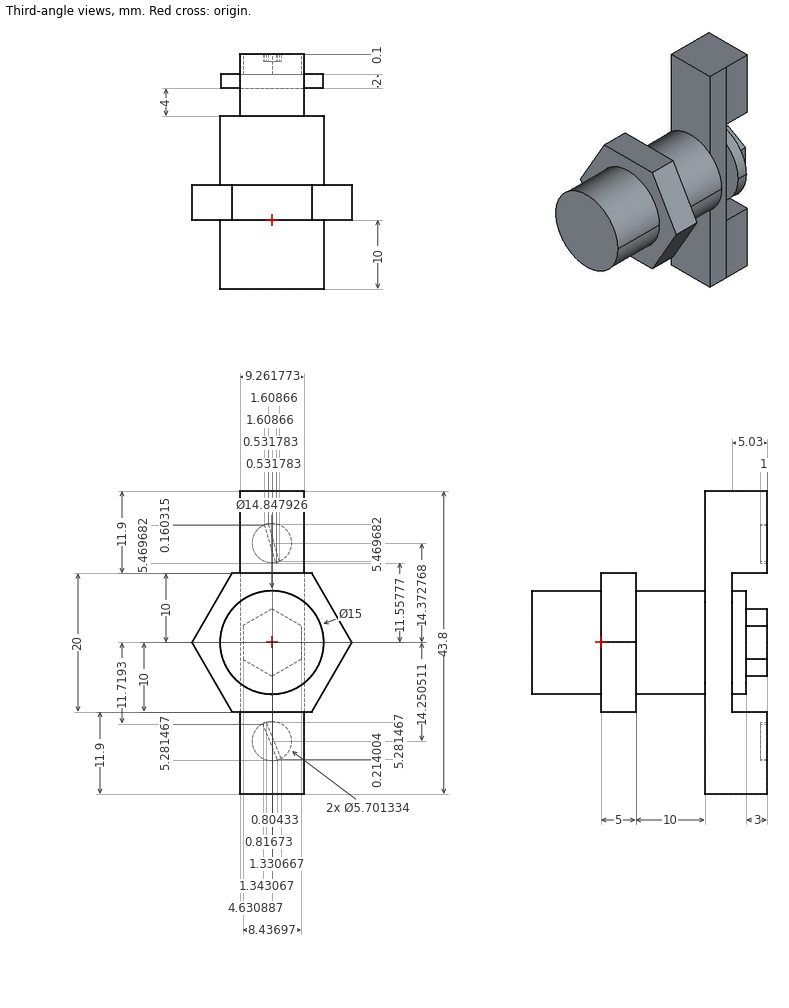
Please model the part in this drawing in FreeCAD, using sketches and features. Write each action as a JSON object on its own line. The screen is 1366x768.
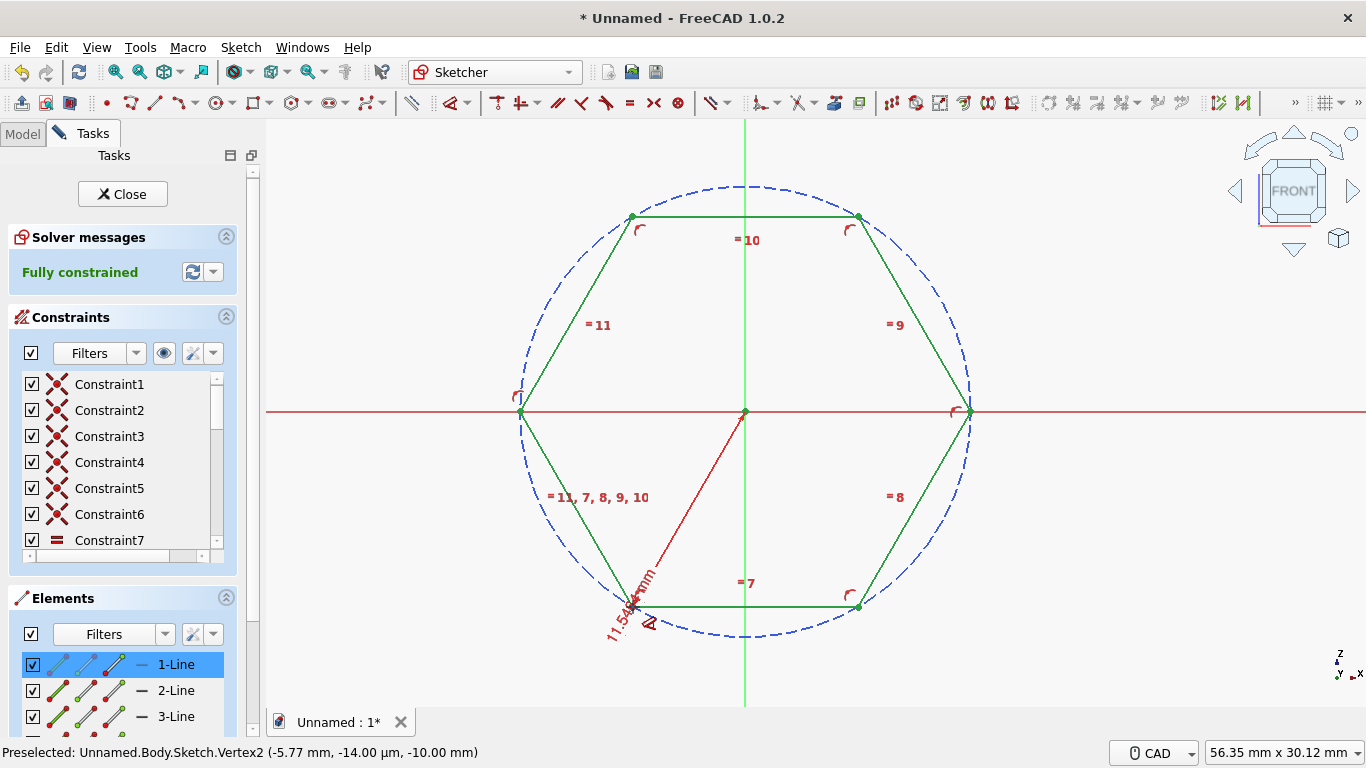
{"action": "left_click", "coordinate": [858, 217]}
{"action": "left_click", "coordinate": [892, 322]}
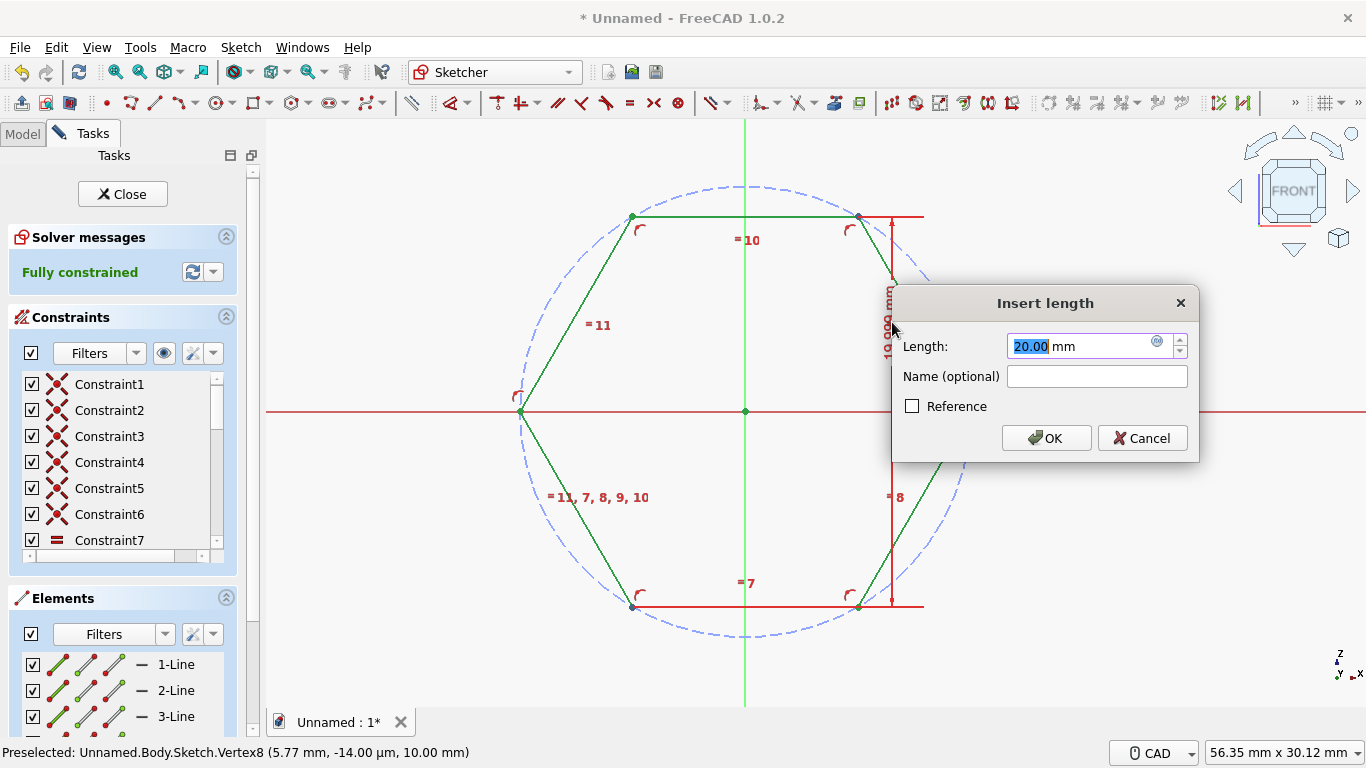
{"action": "type", "text": "20"}
{"action": "key", "text": "Return"}
{"action": "key", "text": "Escape"}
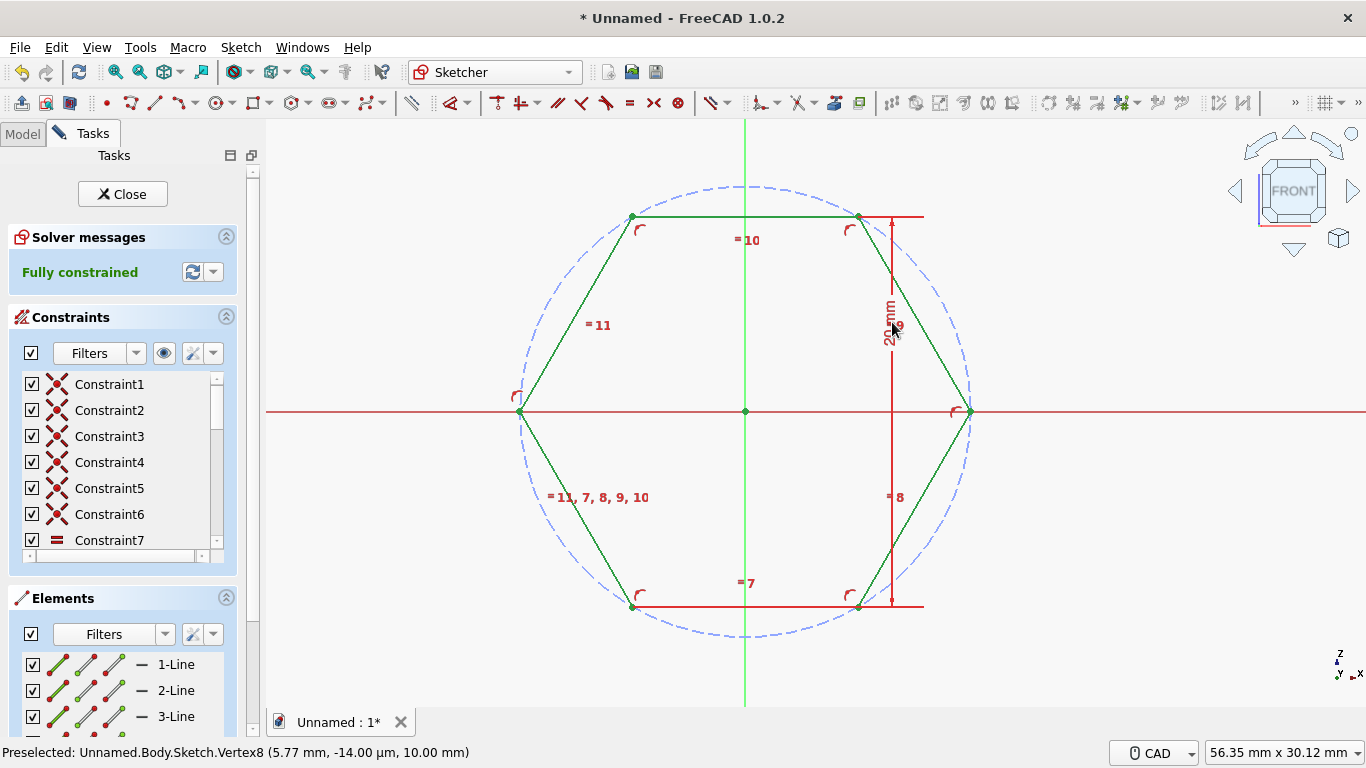
{"action": "left_click", "coordinate": [123, 194]}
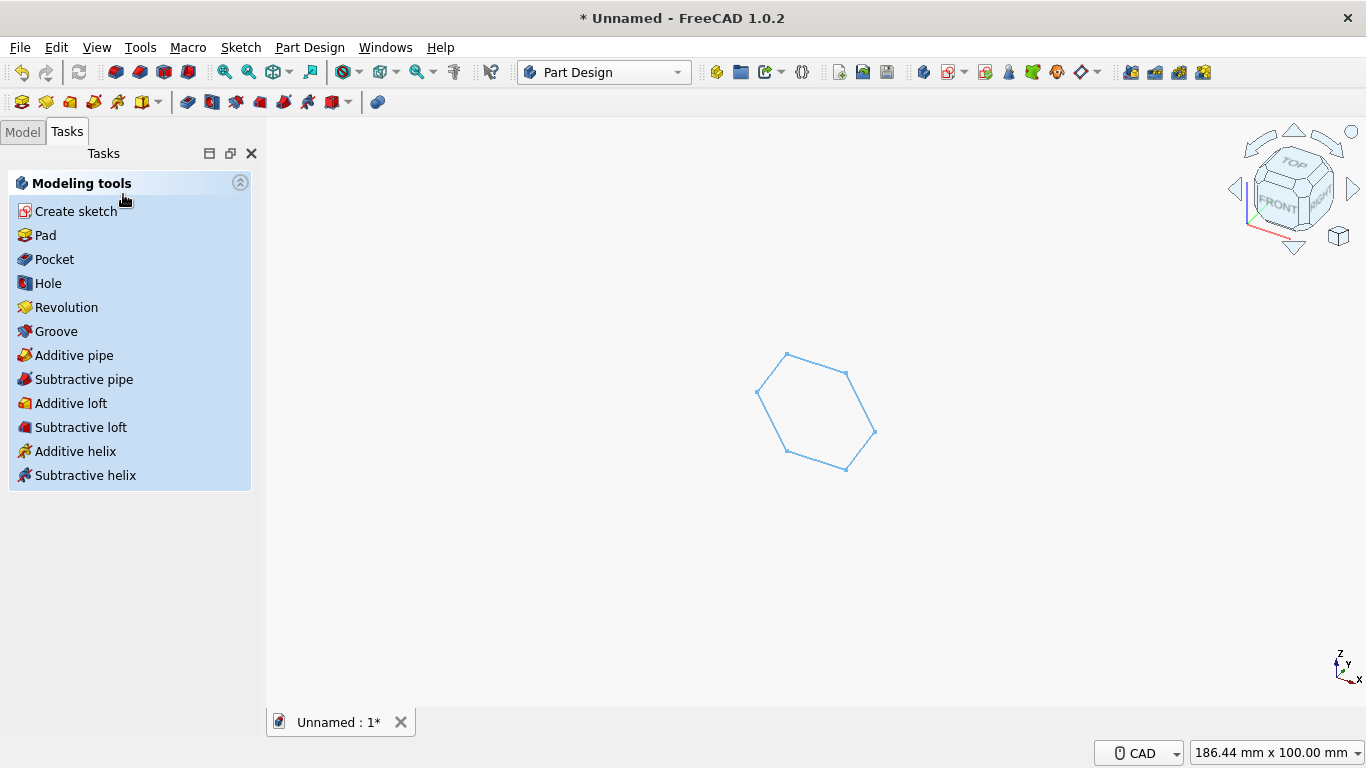
{"action": "left_click", "coordinate": [22, 102]}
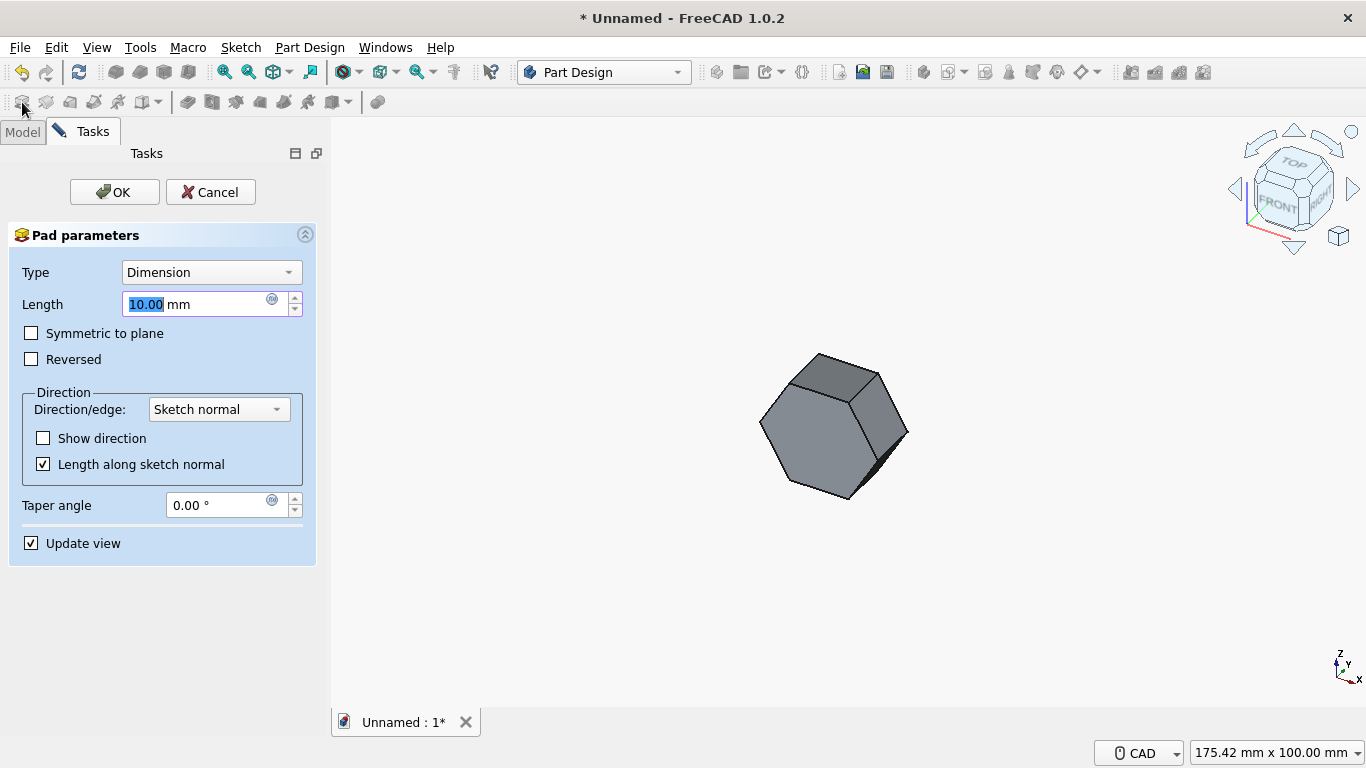
{"action": "type", "text": "5"}
{"action": "key", "text": "Tab"}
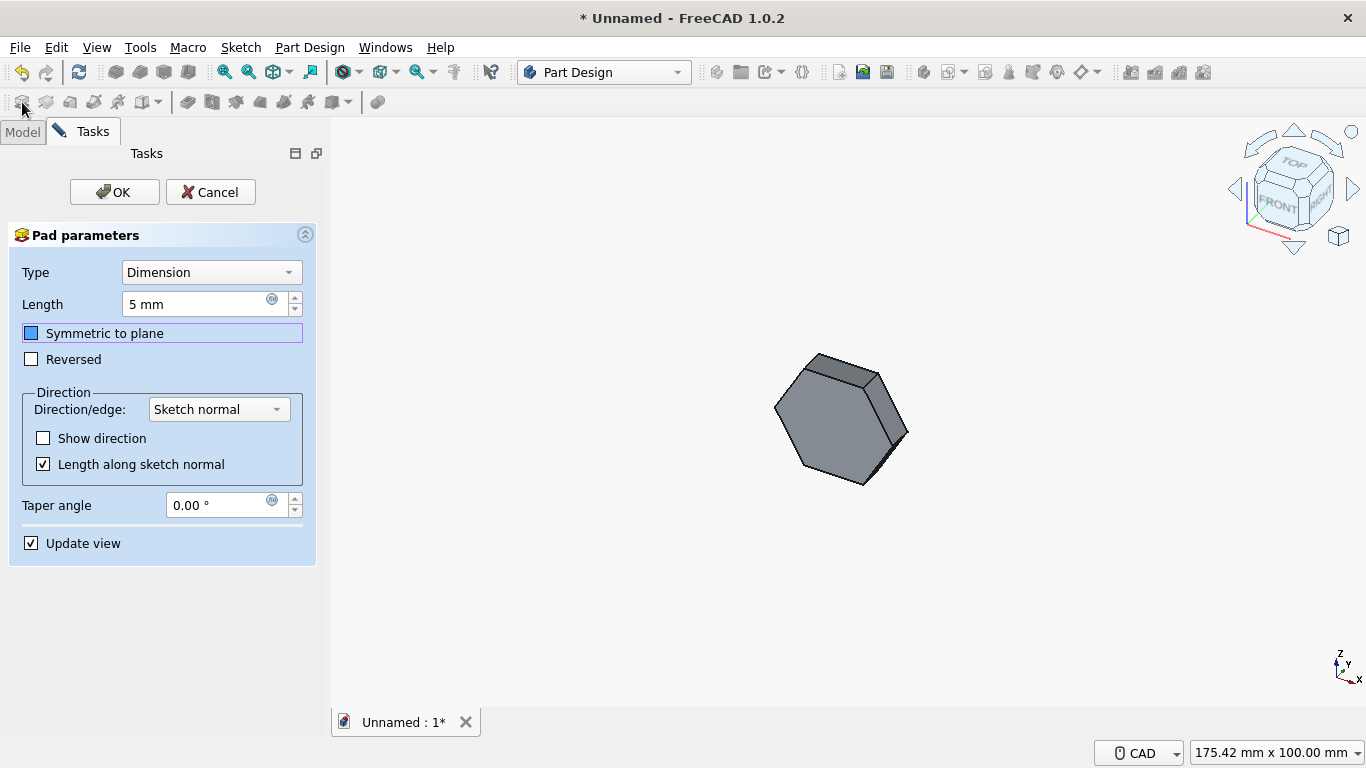
{"action": "left_click", "coordinate": [30, 359]}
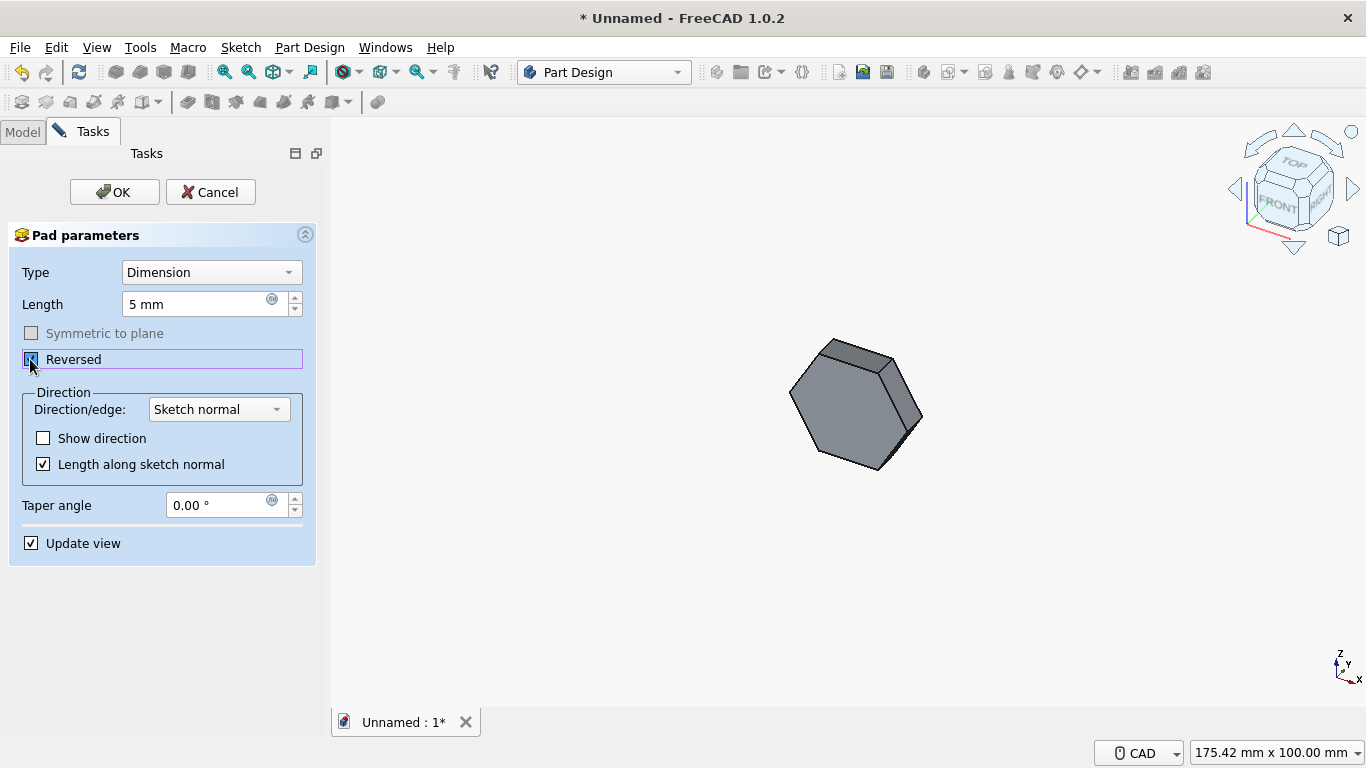
{"action": "left_click", "coordinate": [115, 192]}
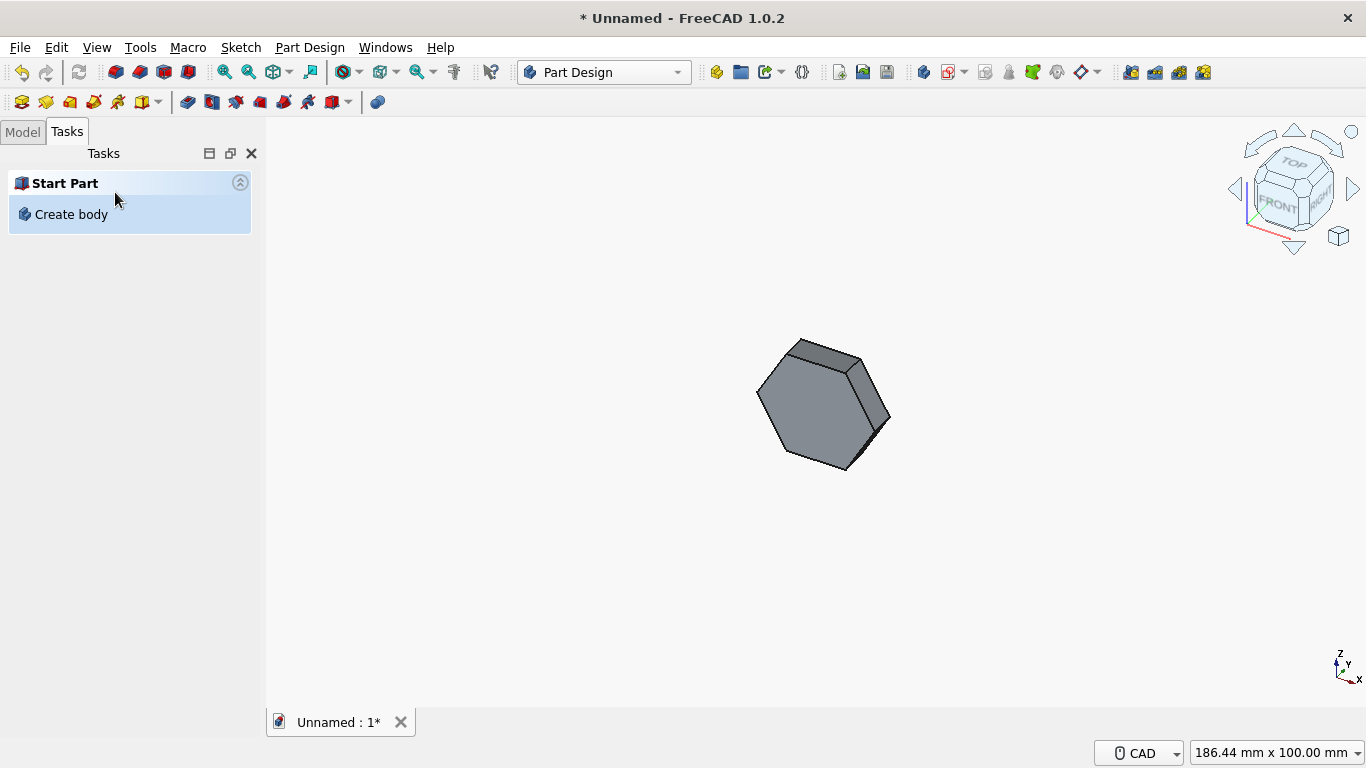
{"action": "left_click", "coordinate": [226, 72]}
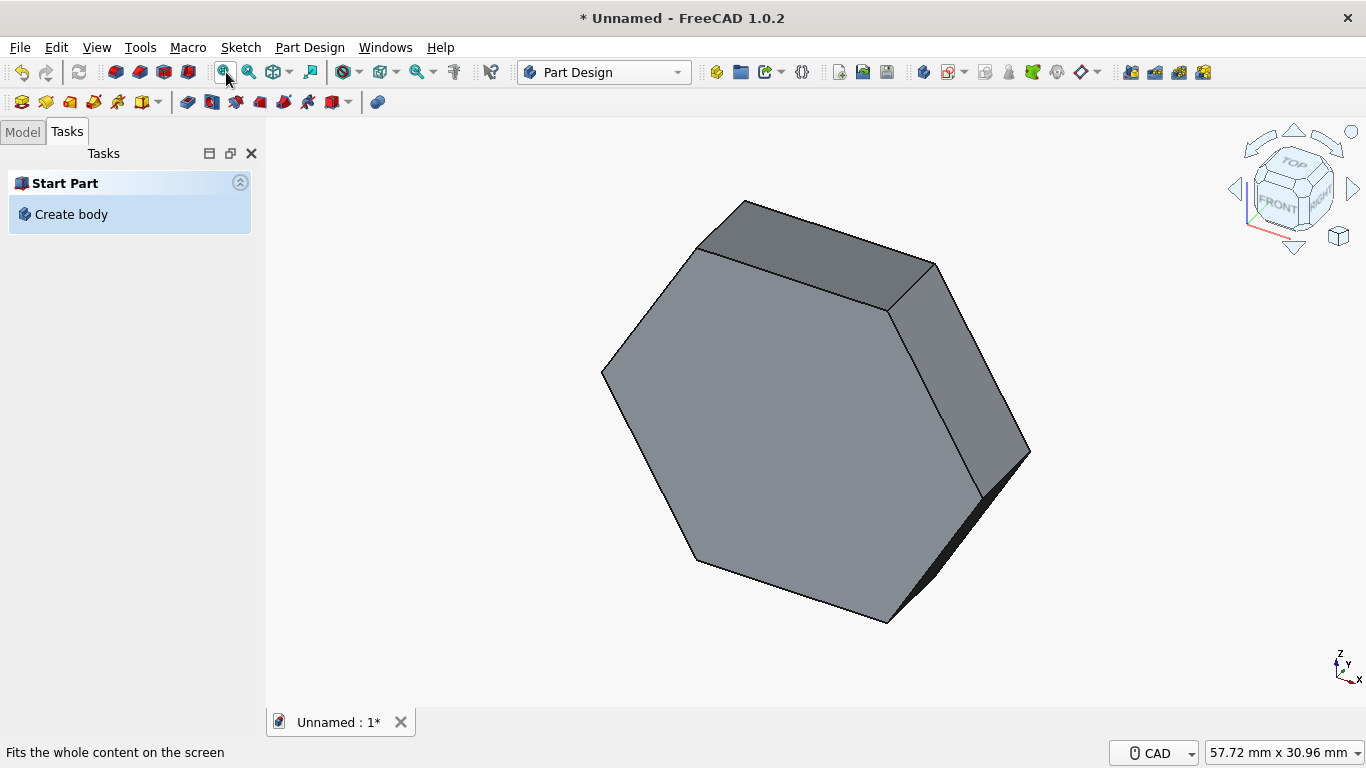
{"action": "left_click", "coordinate": [792, 435]}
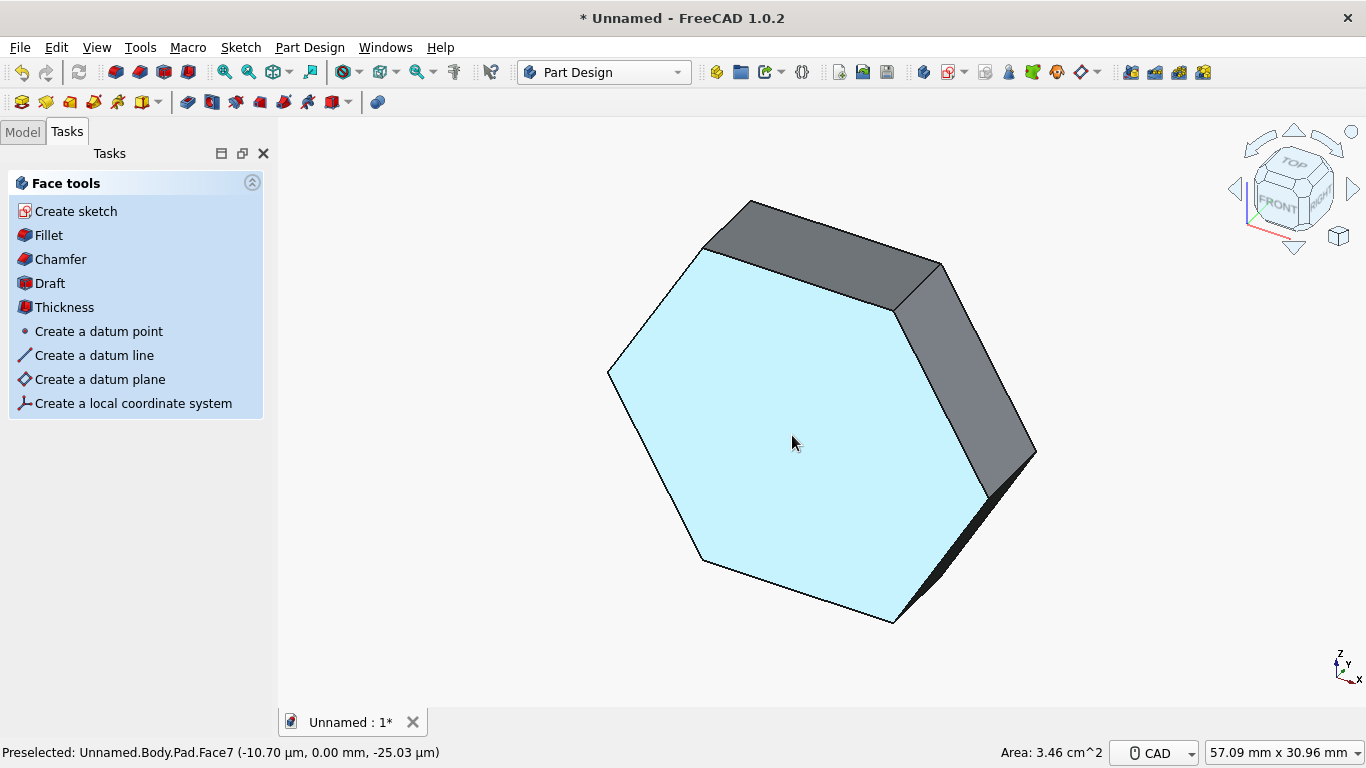
{"action": "left_click", "coordinate": [948, 72]}